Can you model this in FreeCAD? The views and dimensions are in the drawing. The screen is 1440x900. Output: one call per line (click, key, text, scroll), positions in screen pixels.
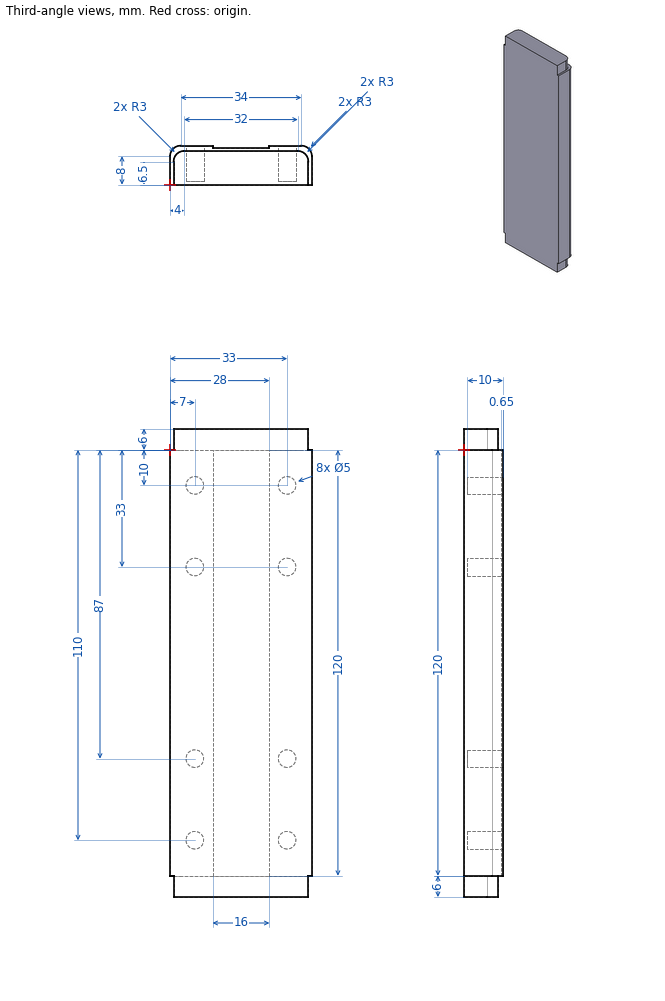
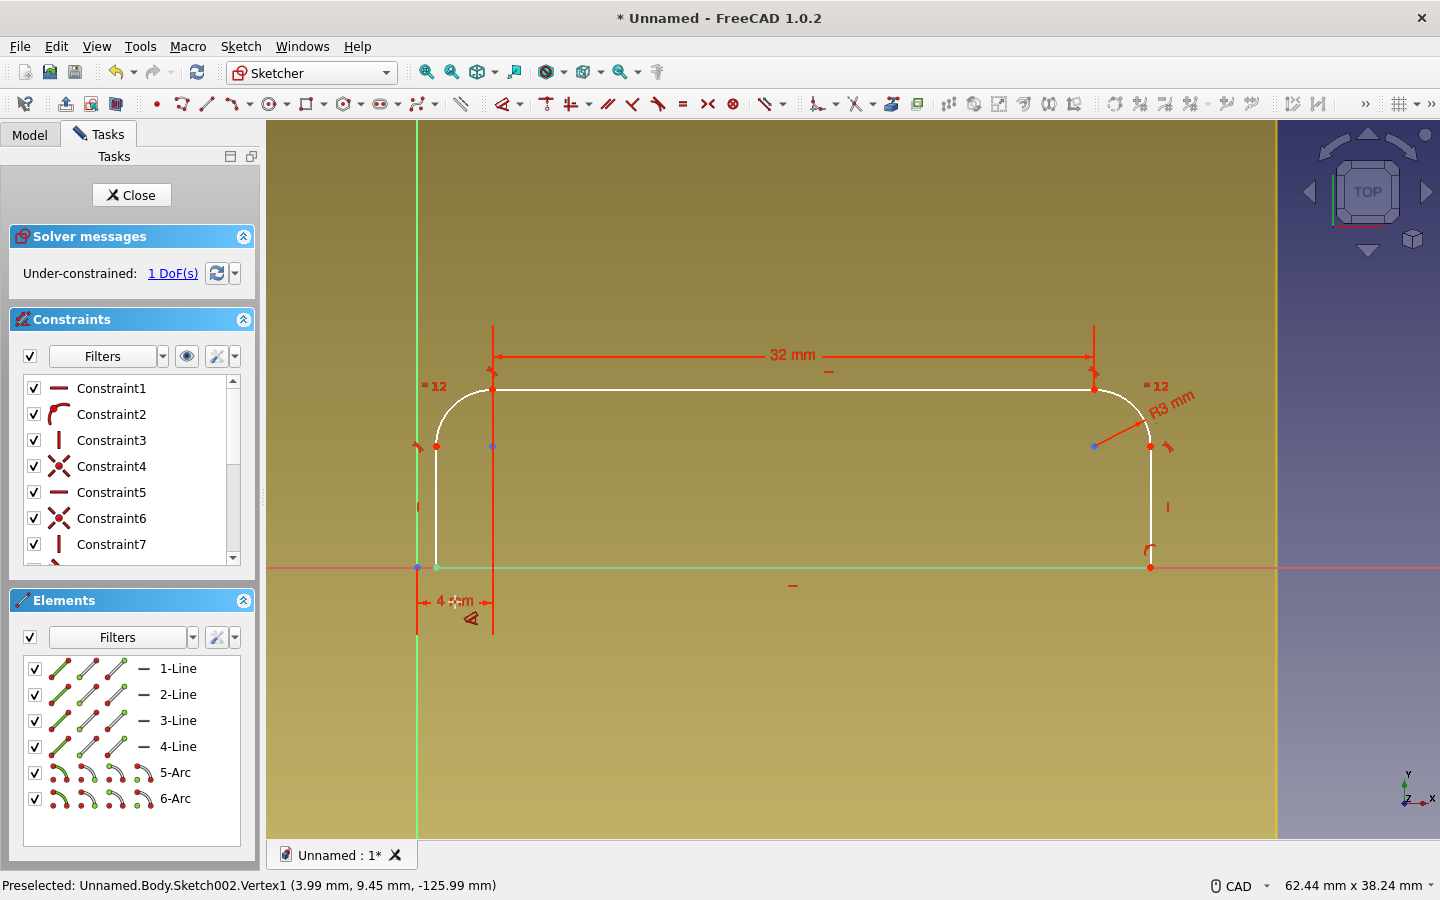
click(1151, 483)
click(1185, 507)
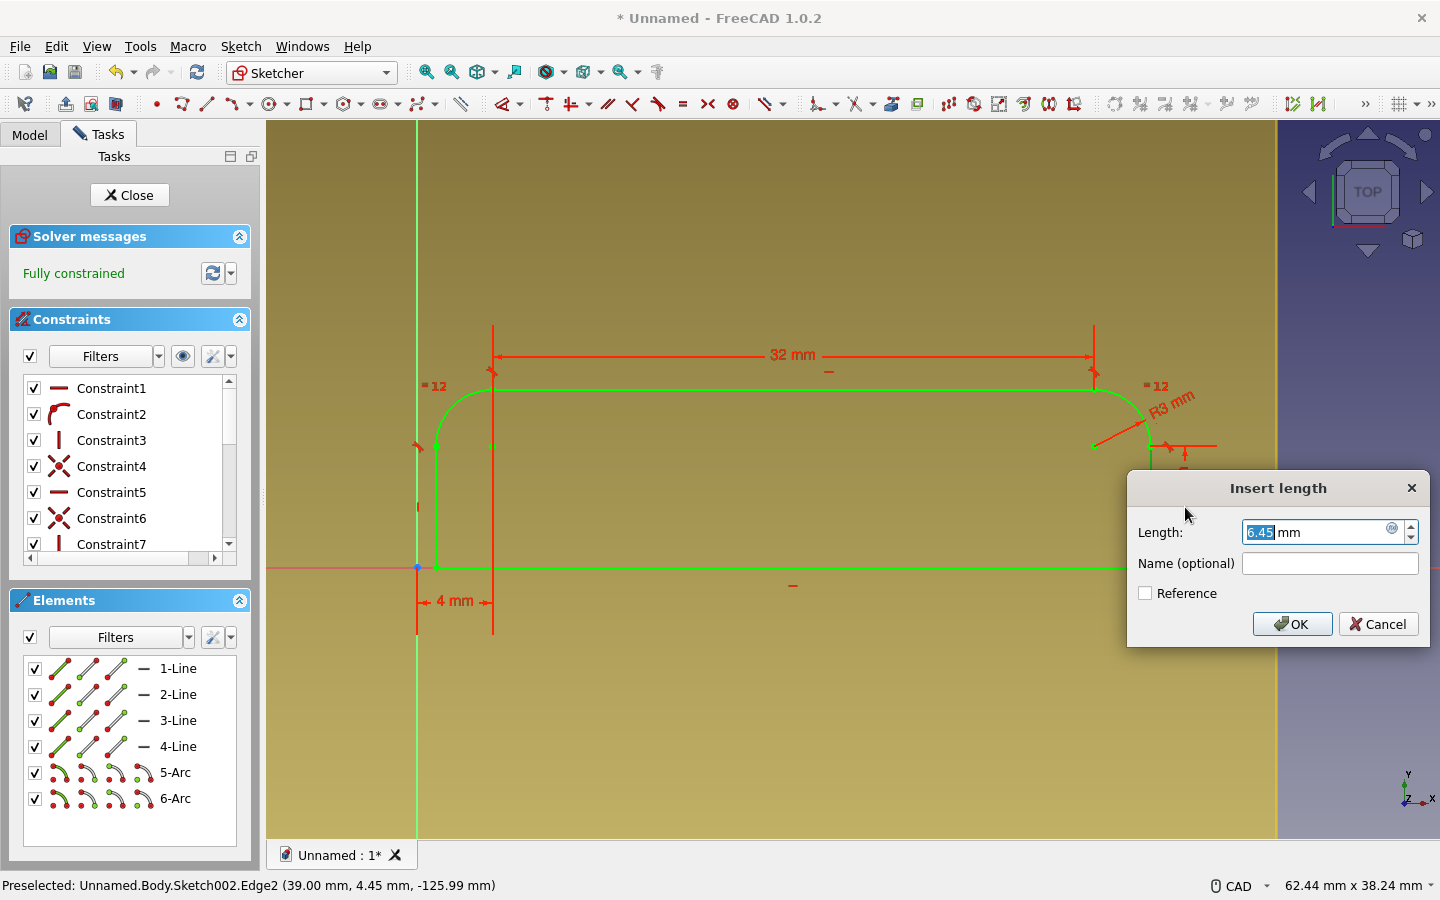
text(6.5)
key(Return)
key(Escape)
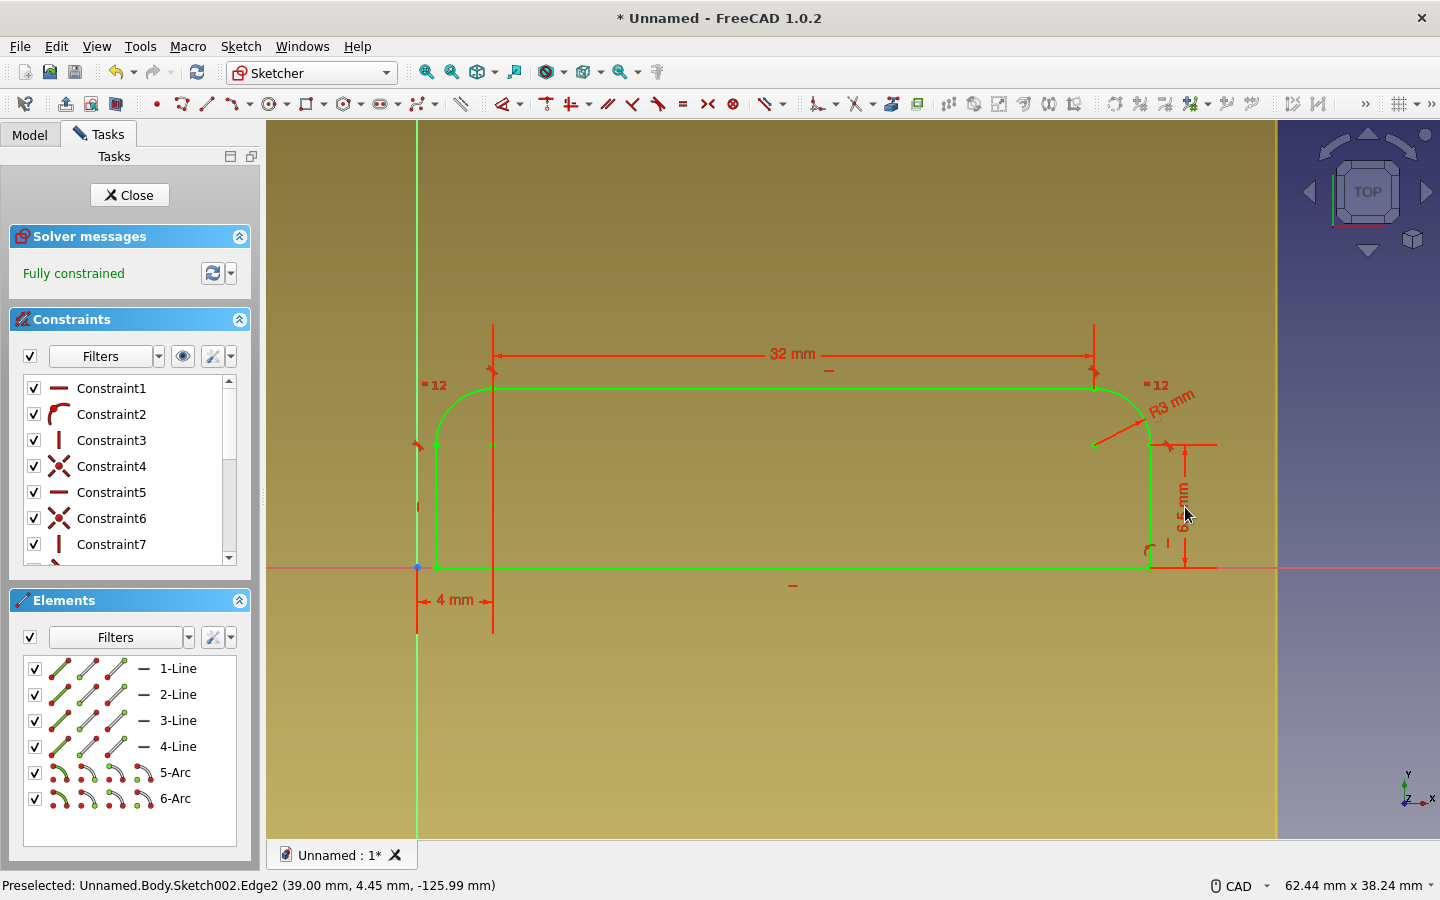
click(130, 195)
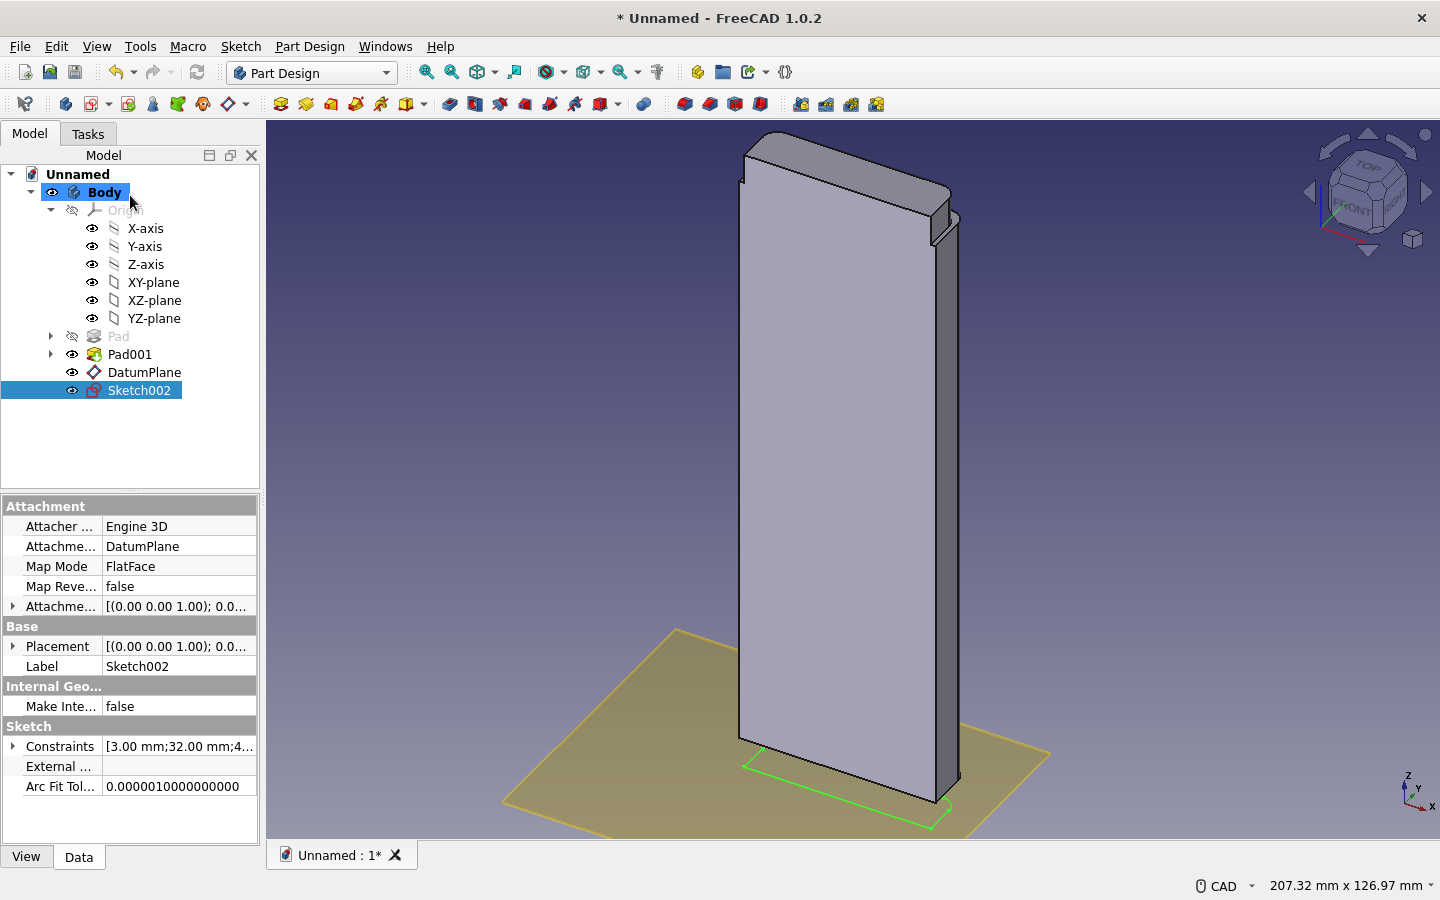
click(281, 104)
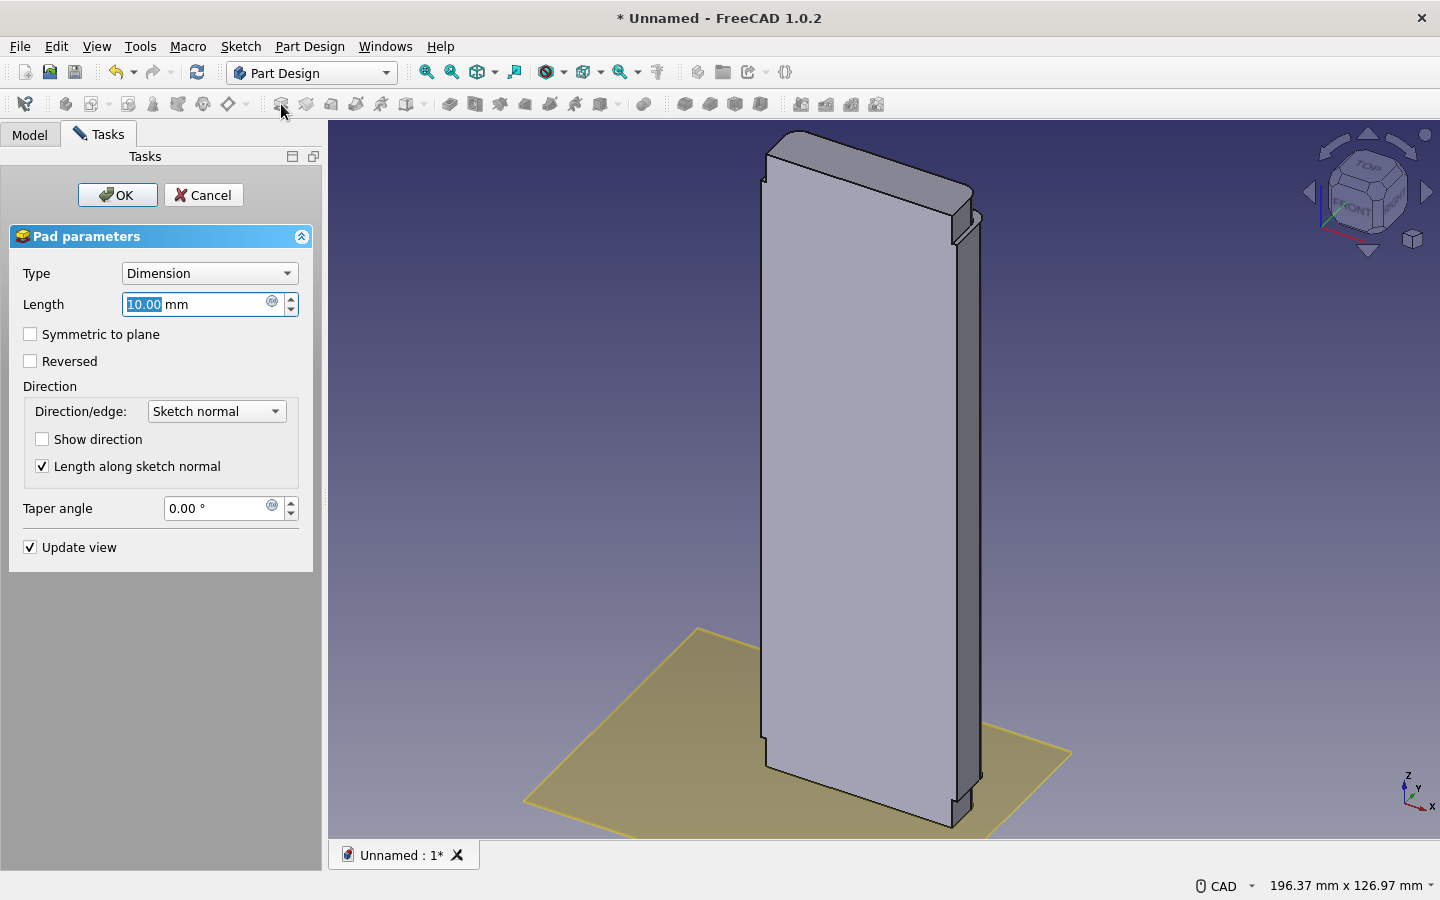
text(6)
key(Tab)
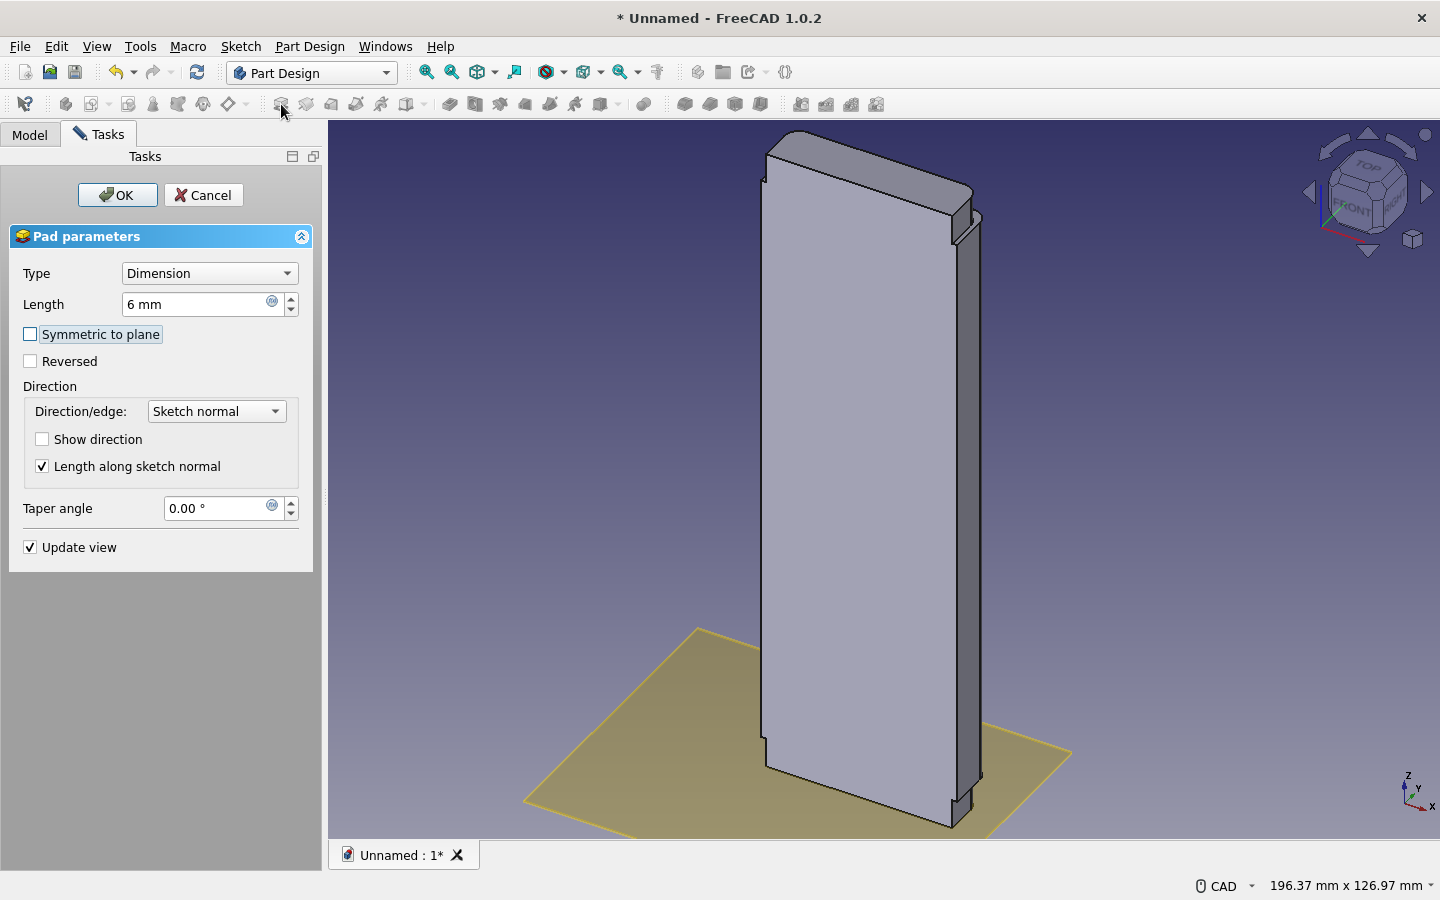
click(118, 195)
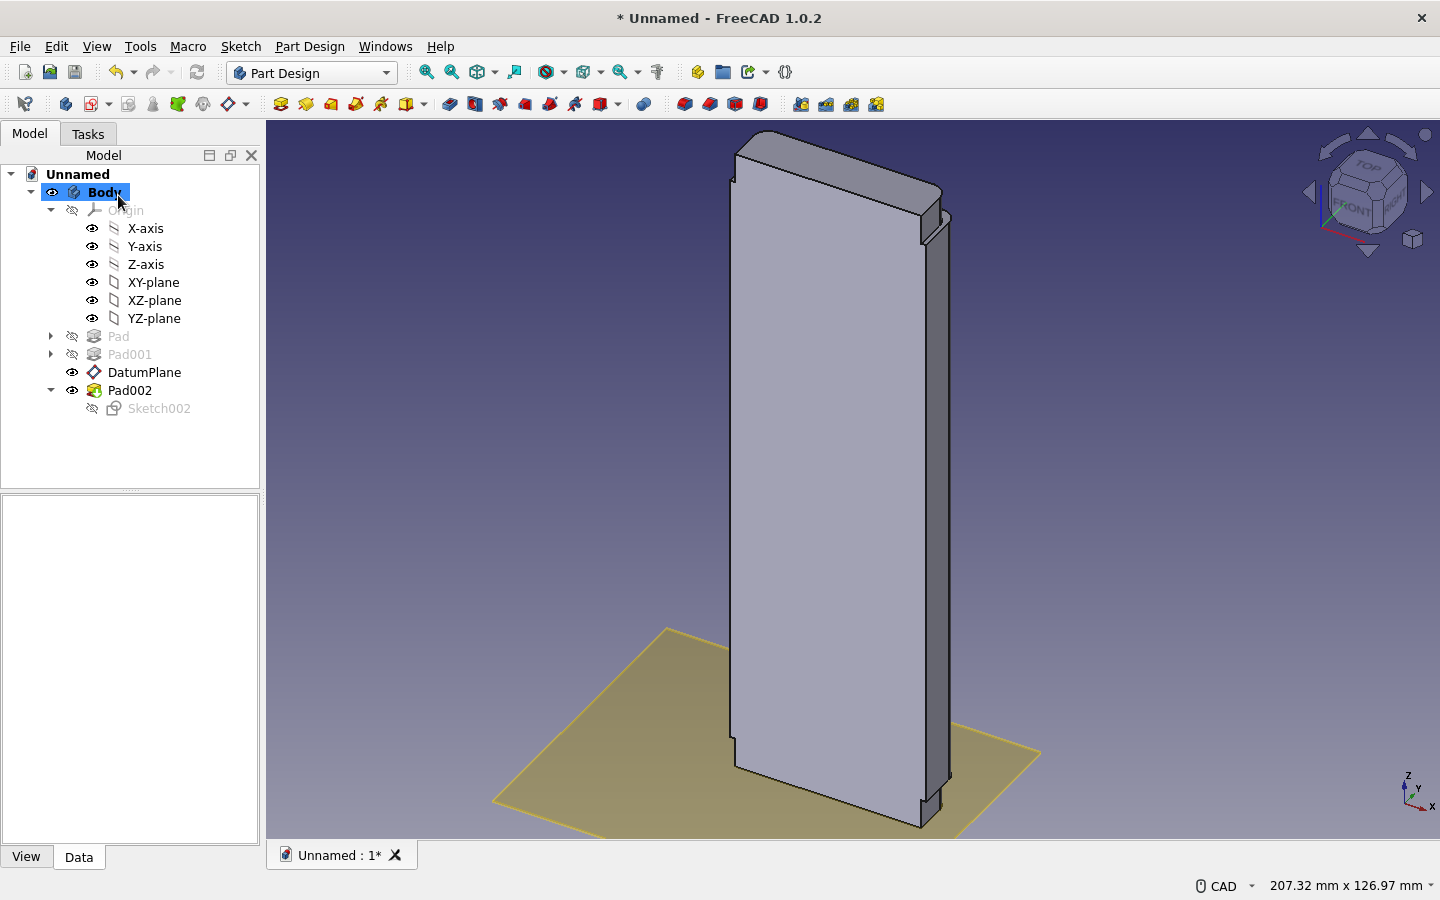
click(117, 372)
key(space)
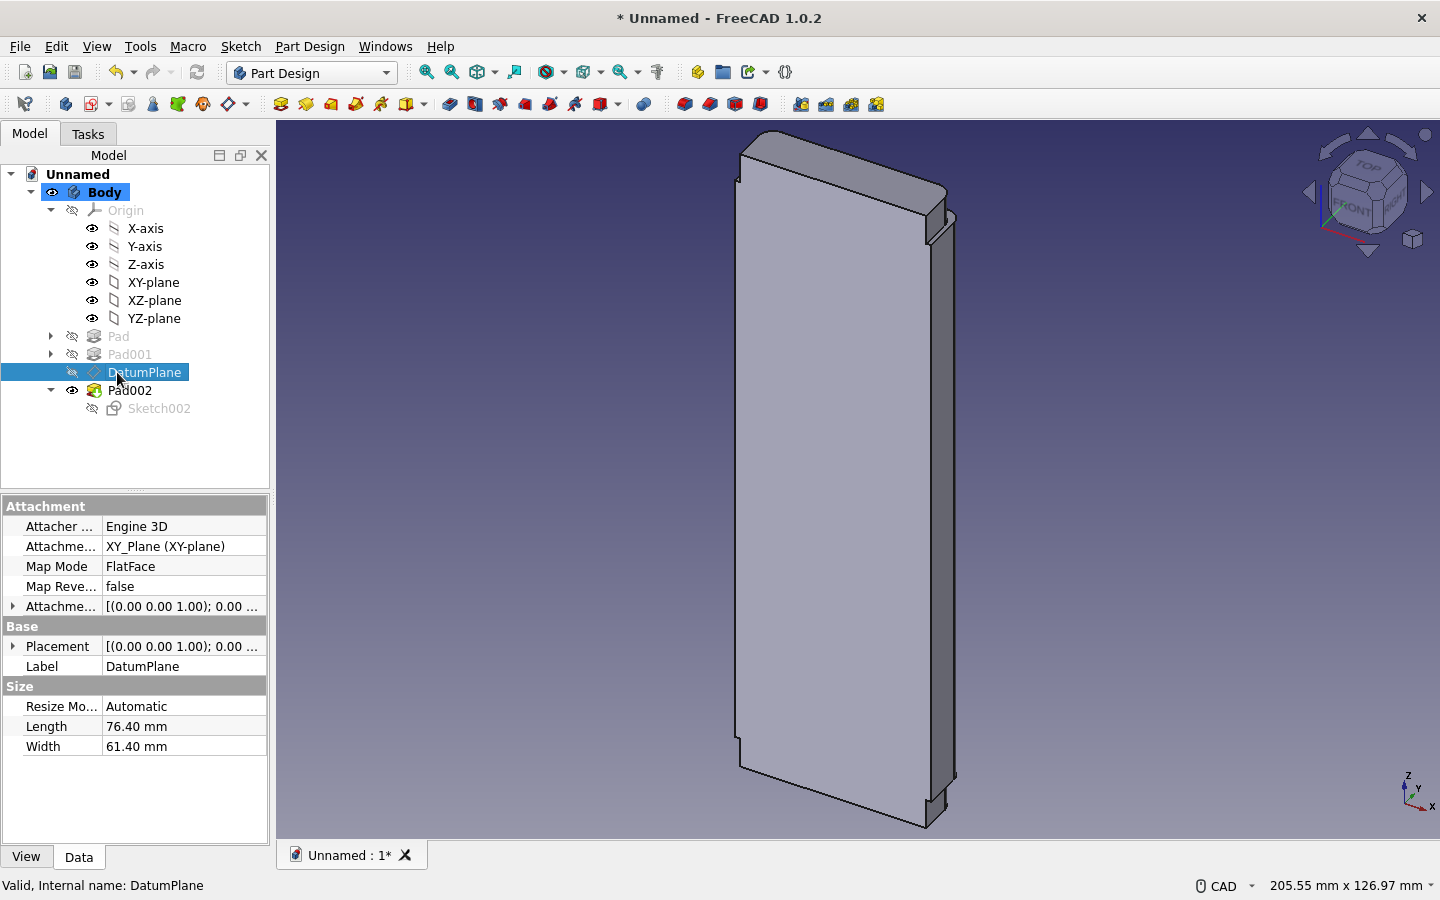
key(4)